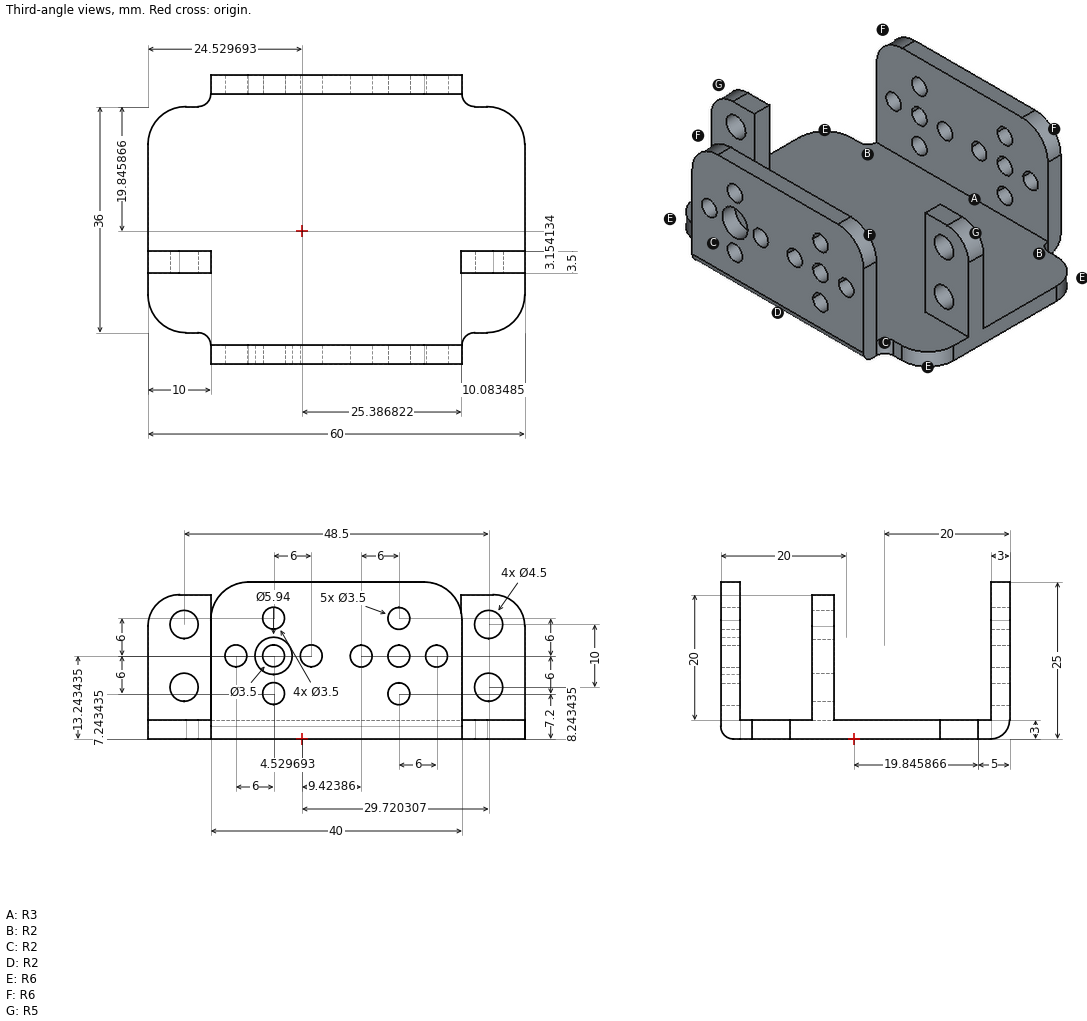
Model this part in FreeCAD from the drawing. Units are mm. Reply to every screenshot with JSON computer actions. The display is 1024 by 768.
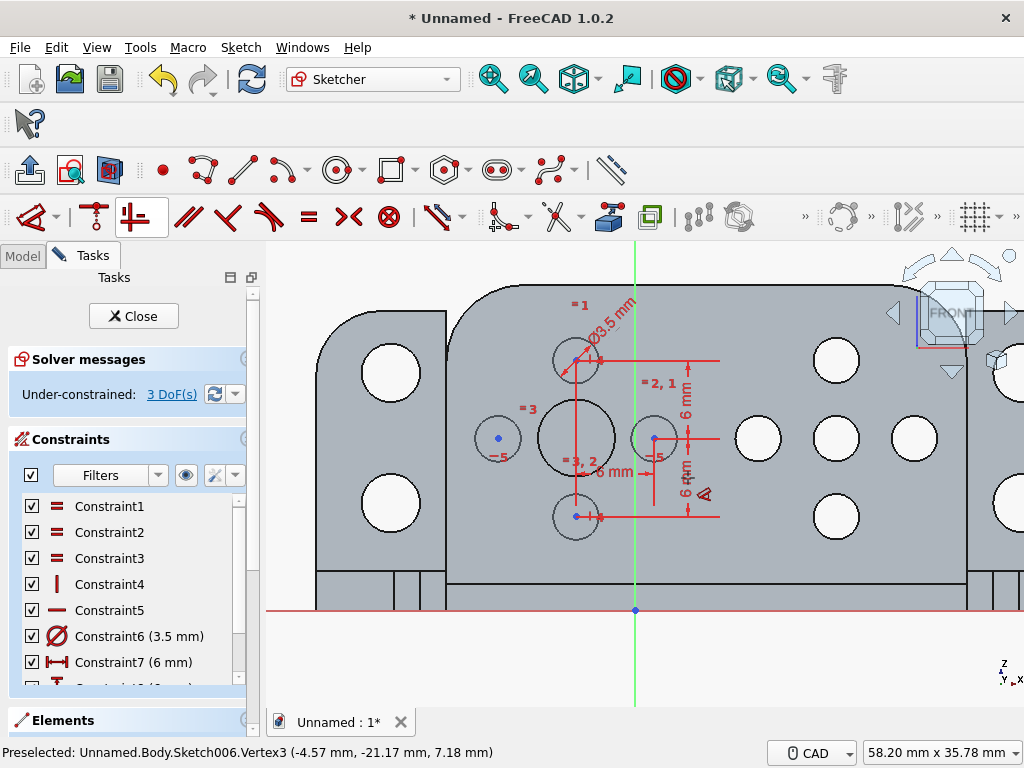
{"action": "left_click", "coordinate": [576, 517]}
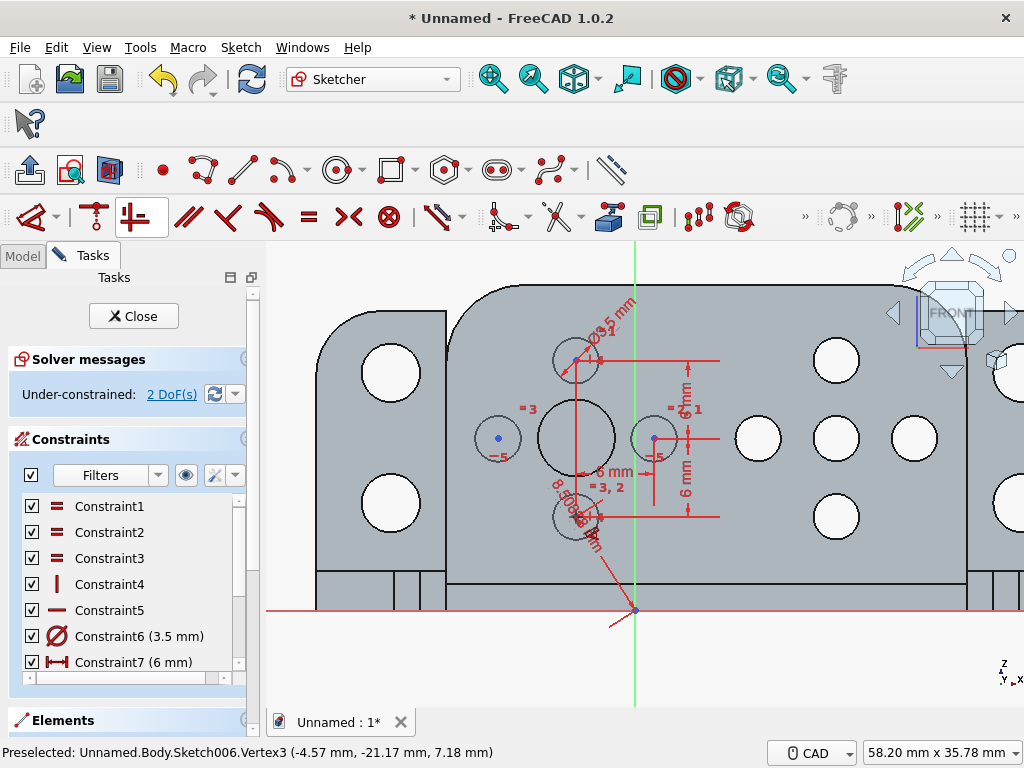
{"action": "left_click", "coordinate": [498, 439]}
{"action": "left_click", "coordinate": [537, 551]}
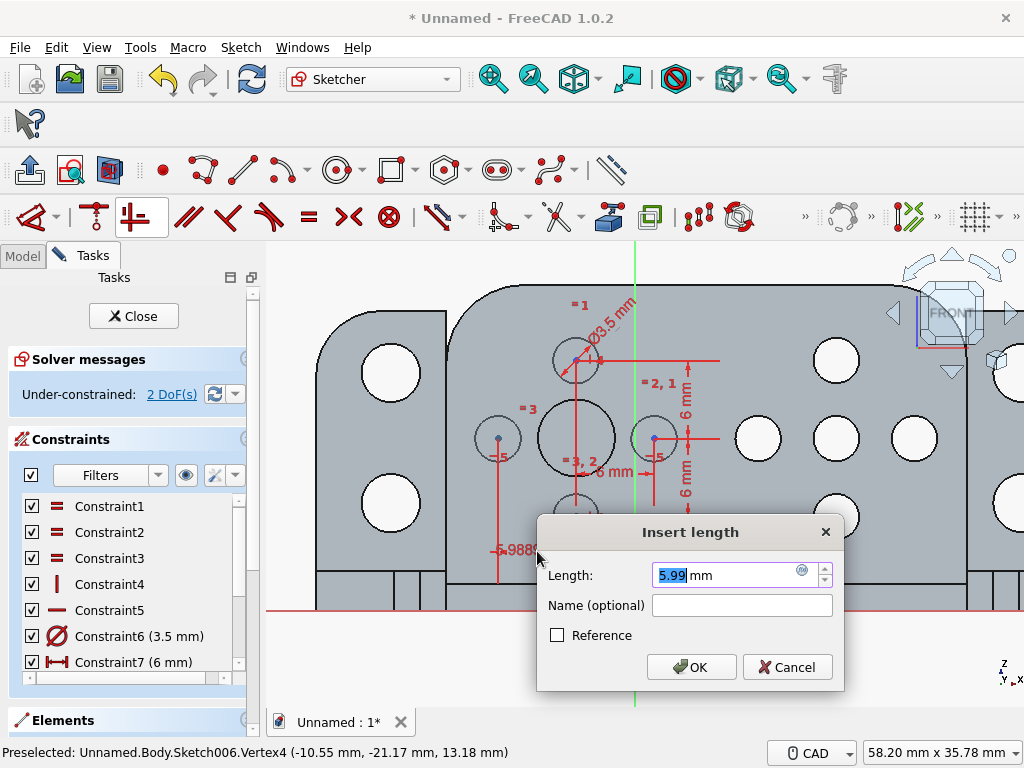
{"action": "type", "text": "6"}
{"action": "key", "text": "Return"}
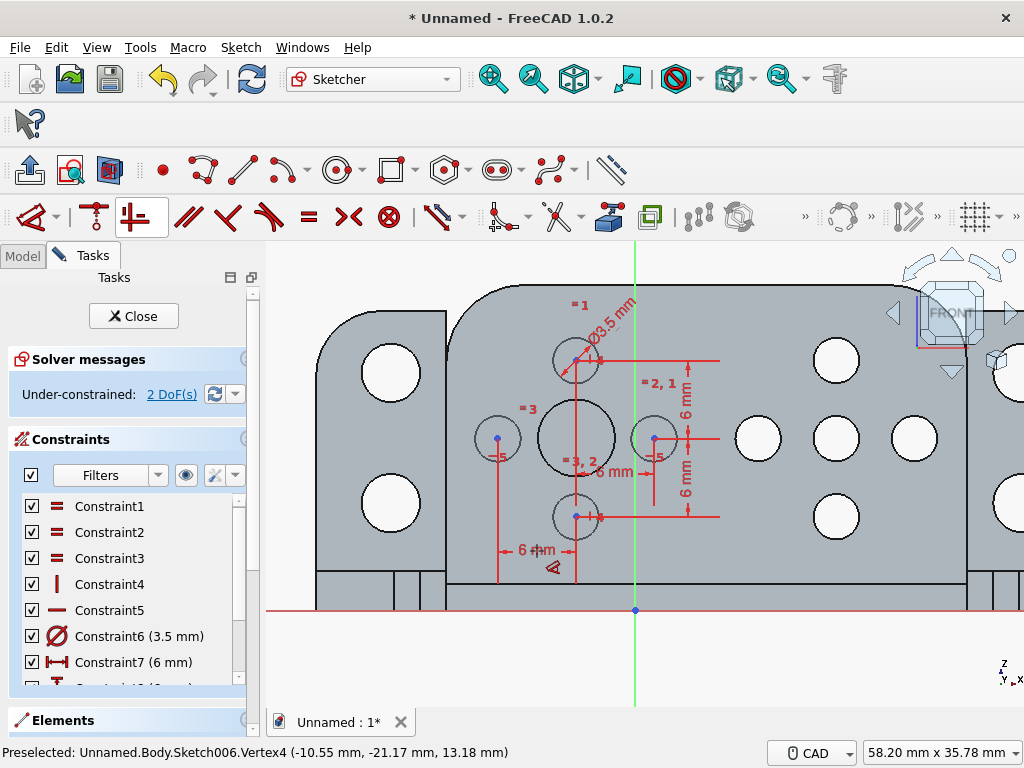
{"action": "left_click", "coordinate": [576, 361]}
{"action": "left_click", "coordinate": [606, 645]}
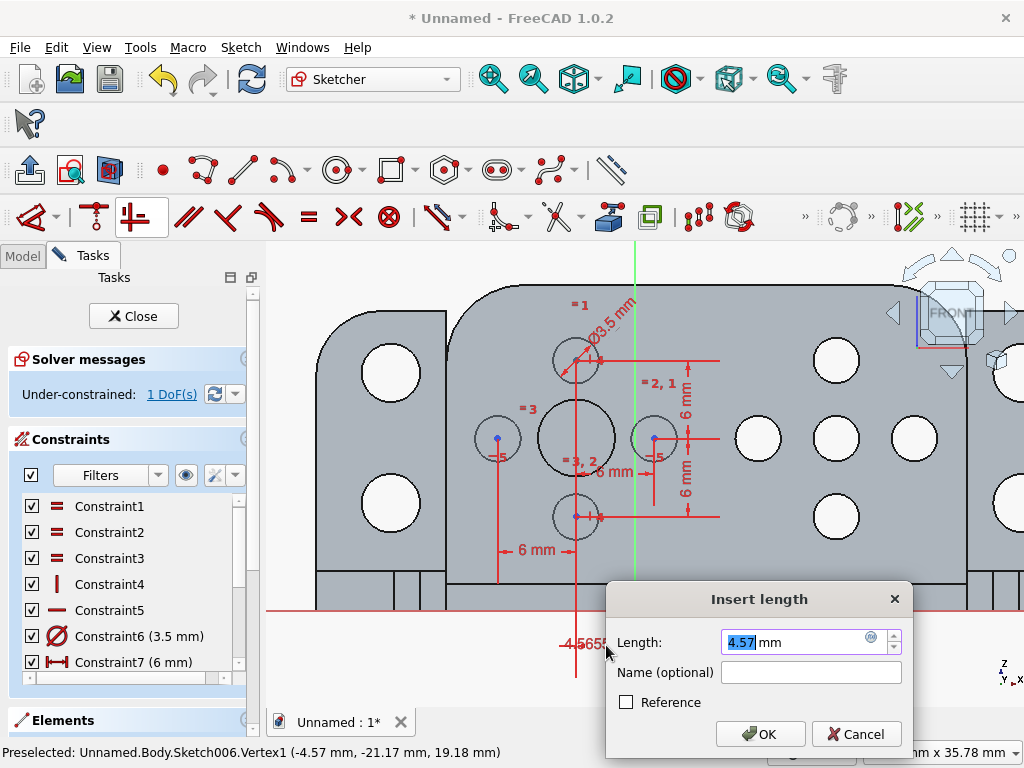
{"action": "type", "text": "4.529693"}
{"action": "key", "text": "Return"}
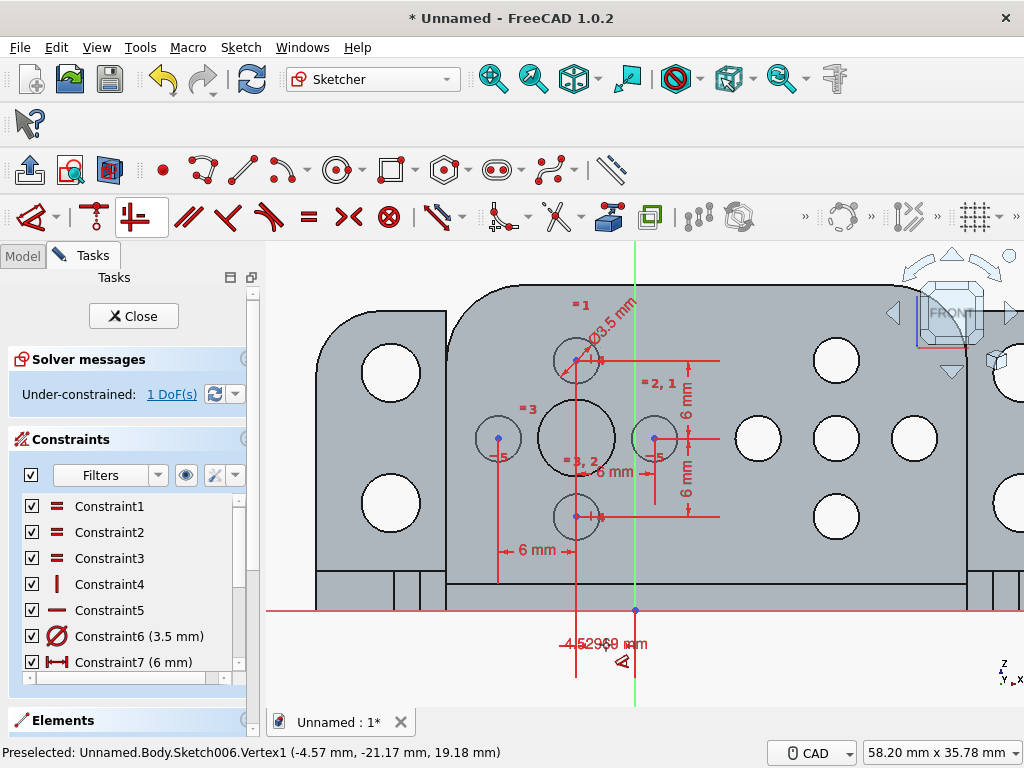
{"action": "left_click", "coordinate": [576, 517]}
{"action": "left_click", "coordinate": [669, 564]}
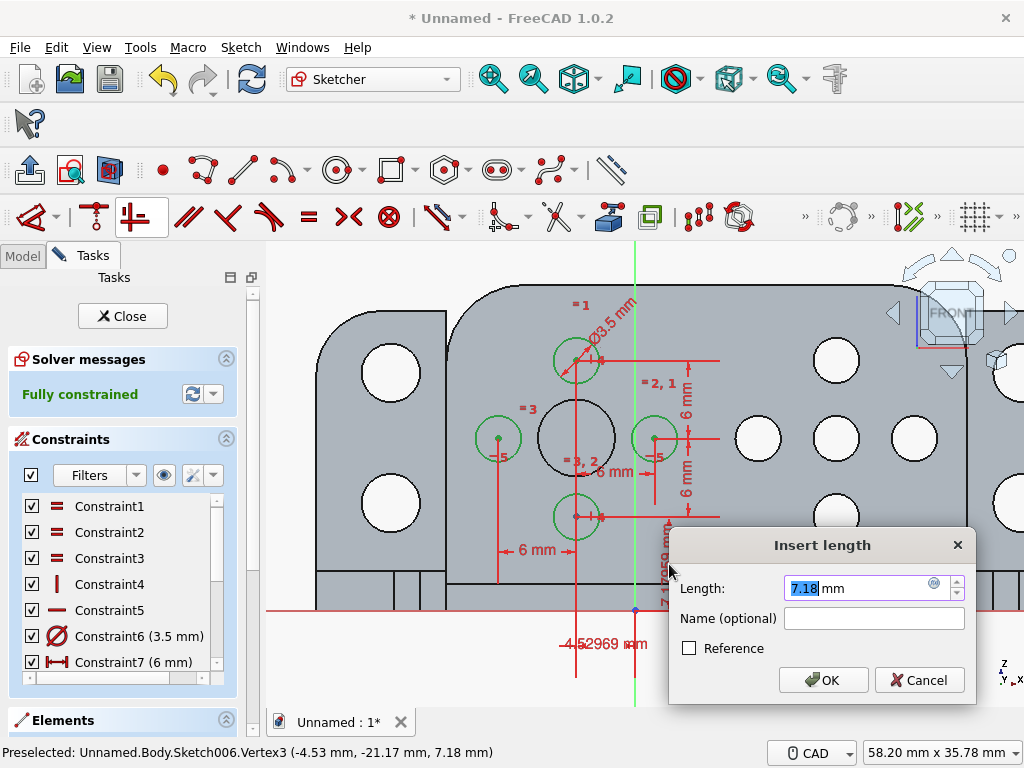
{"action": "type", "text": "7.243435"}
{"action": "key", "text": "Return"}
{"action": "key", "text": "Escape"}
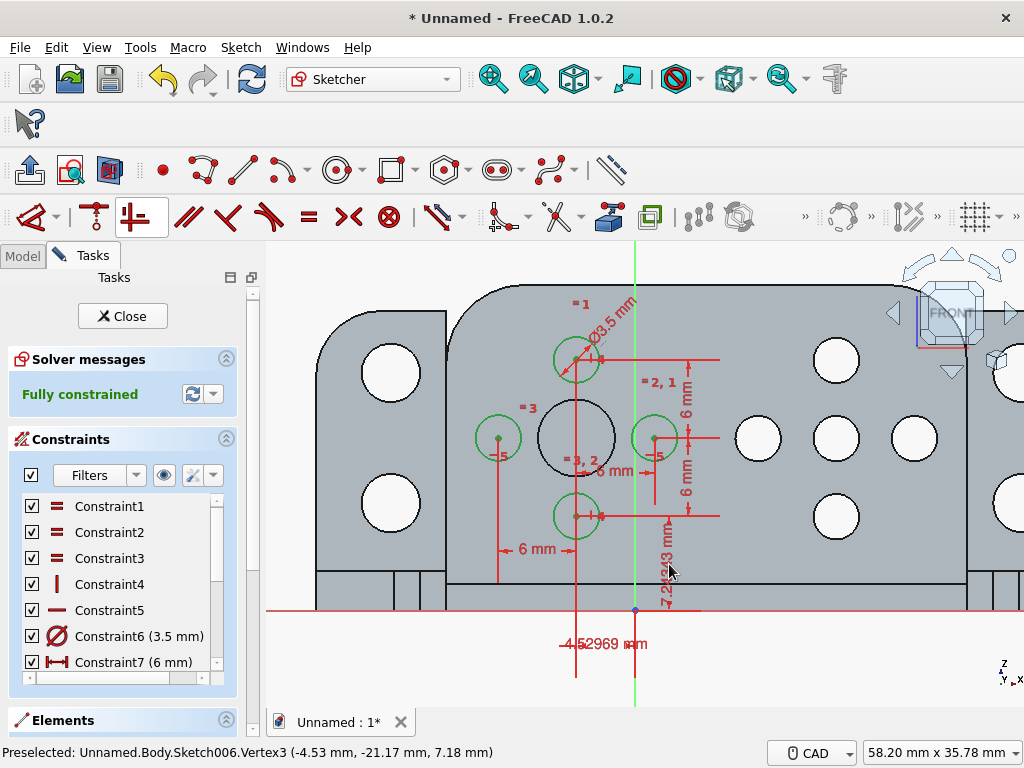
{"action": "left_click", "coordinate": [123, 316]}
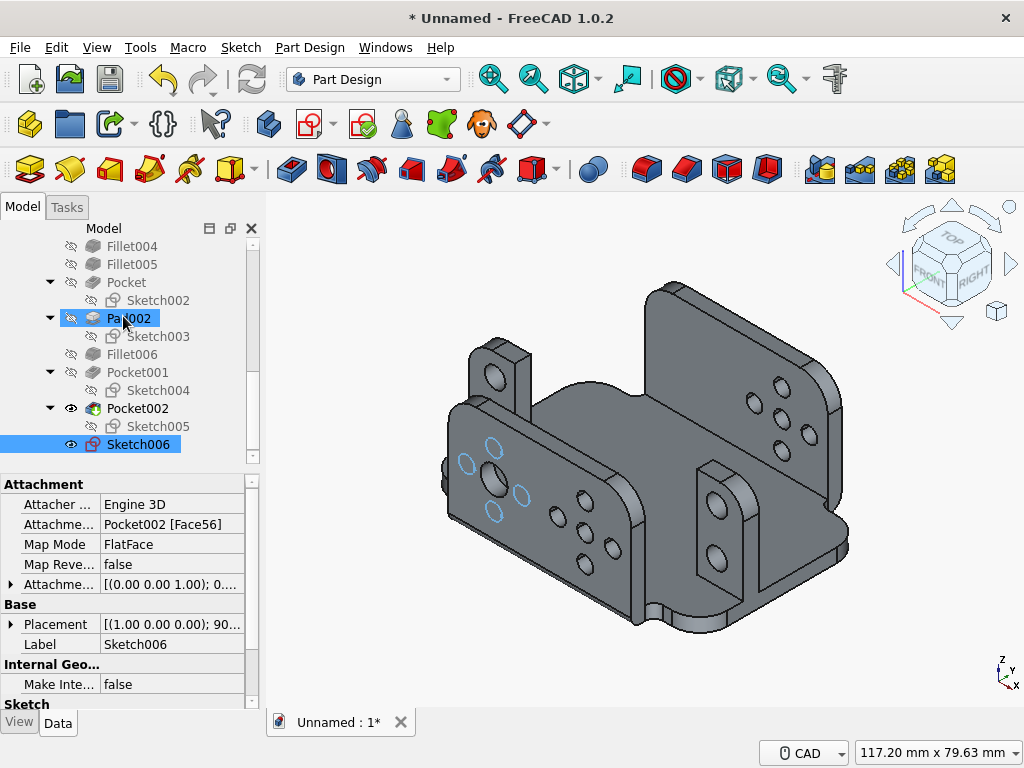
{"action": "left_click", "coordinate": [292, 170]}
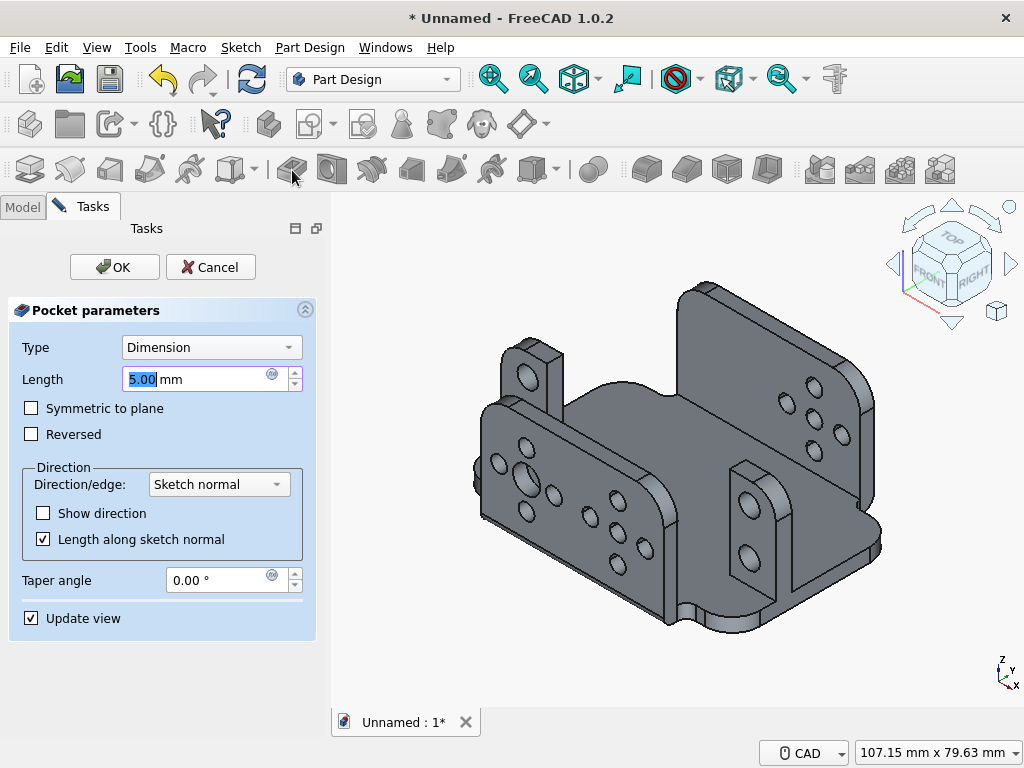
{"action": "left_click", "coordinate": [212, 348]}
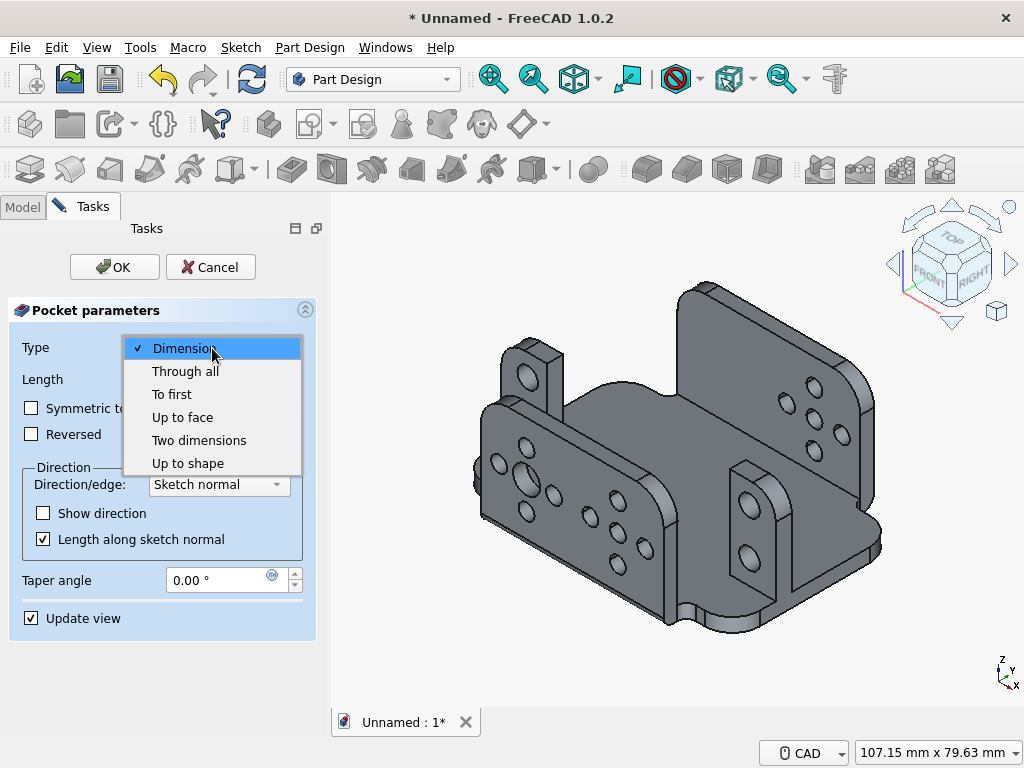
{"action": "left_click", "coordinate": [212, 372]}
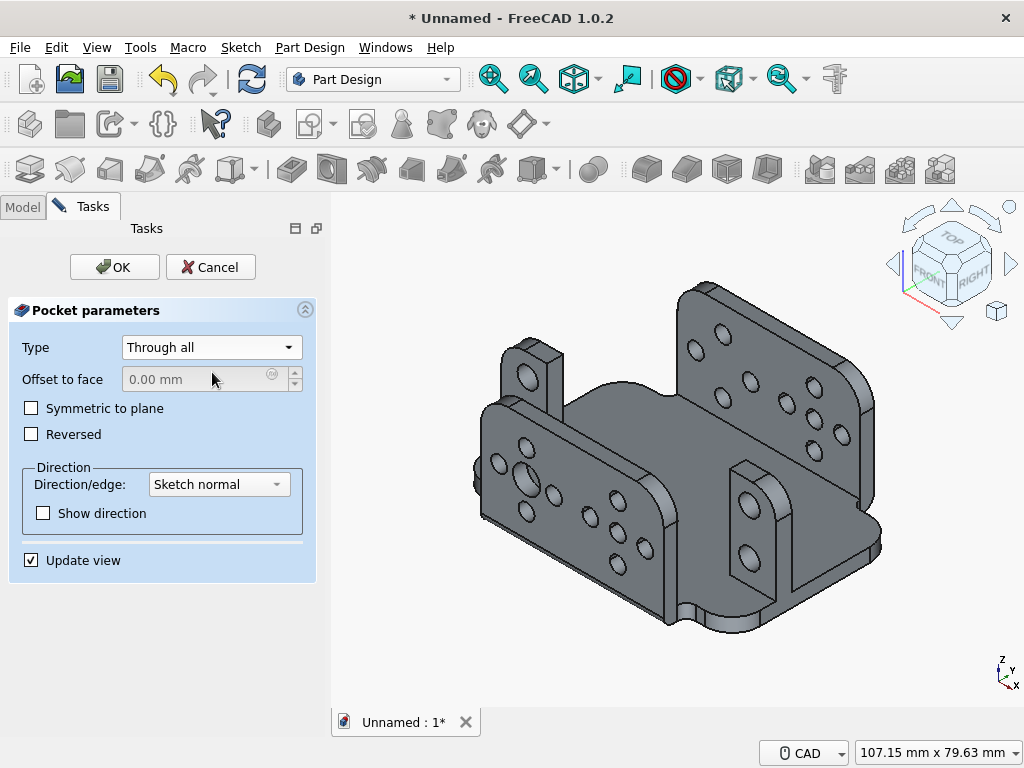
{"action": "left_click", "coordinate": [115, 267]}